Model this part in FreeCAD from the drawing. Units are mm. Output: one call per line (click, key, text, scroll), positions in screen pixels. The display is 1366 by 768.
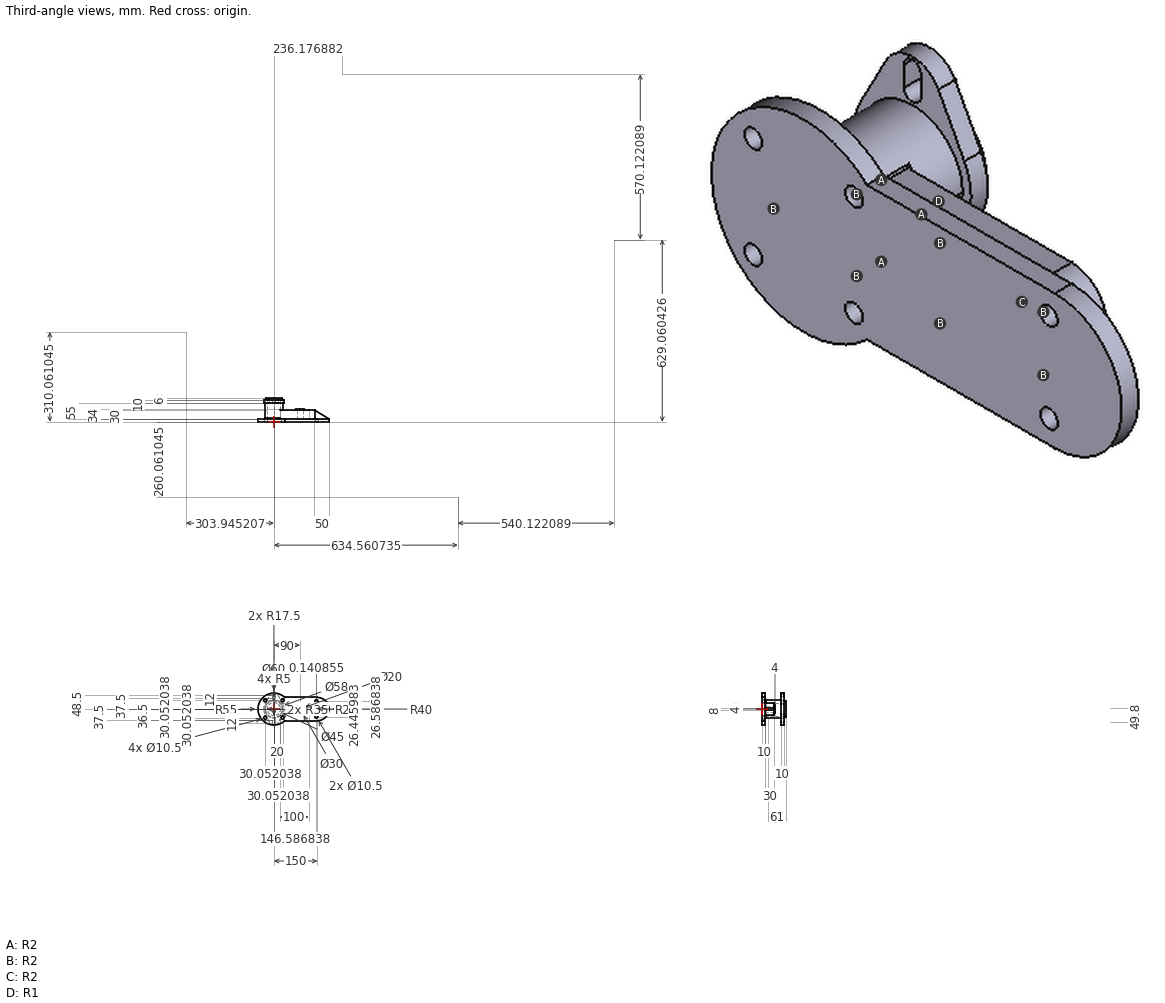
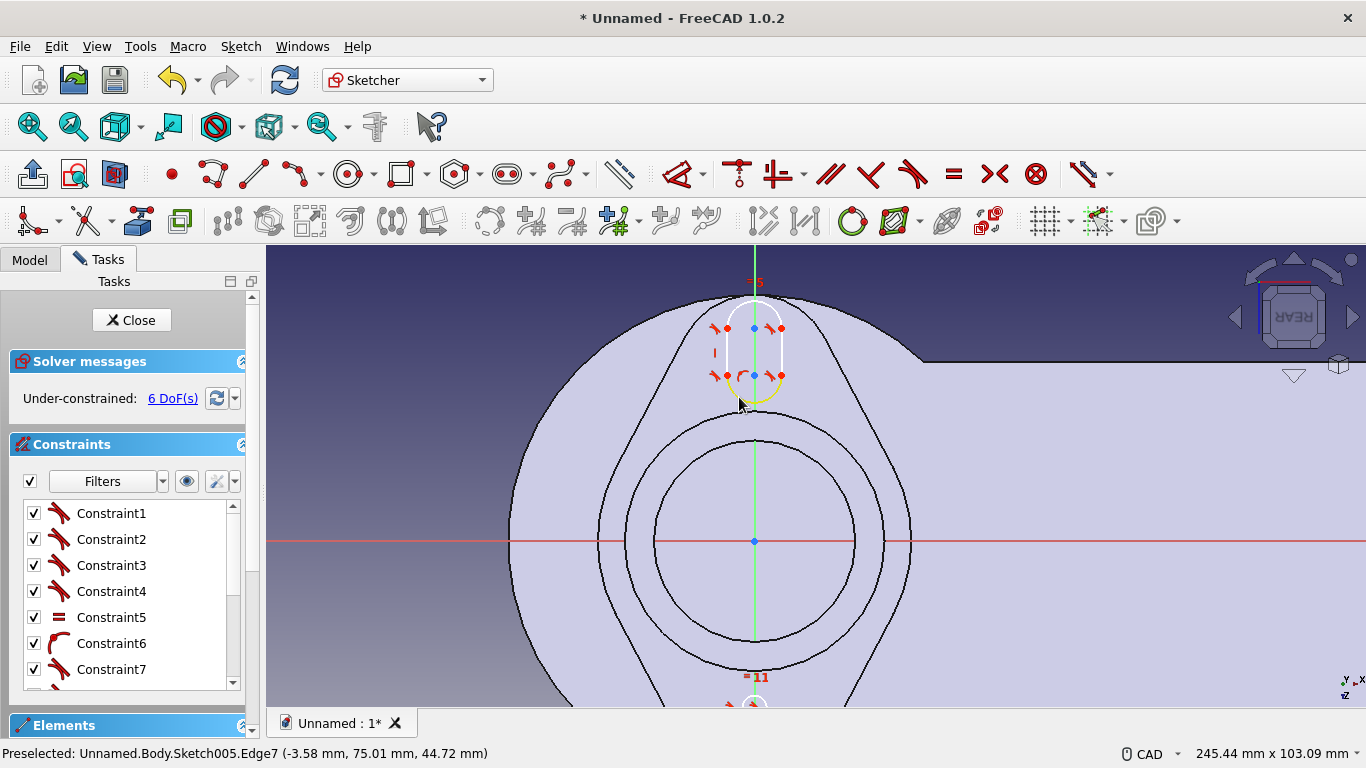
click(739, 398)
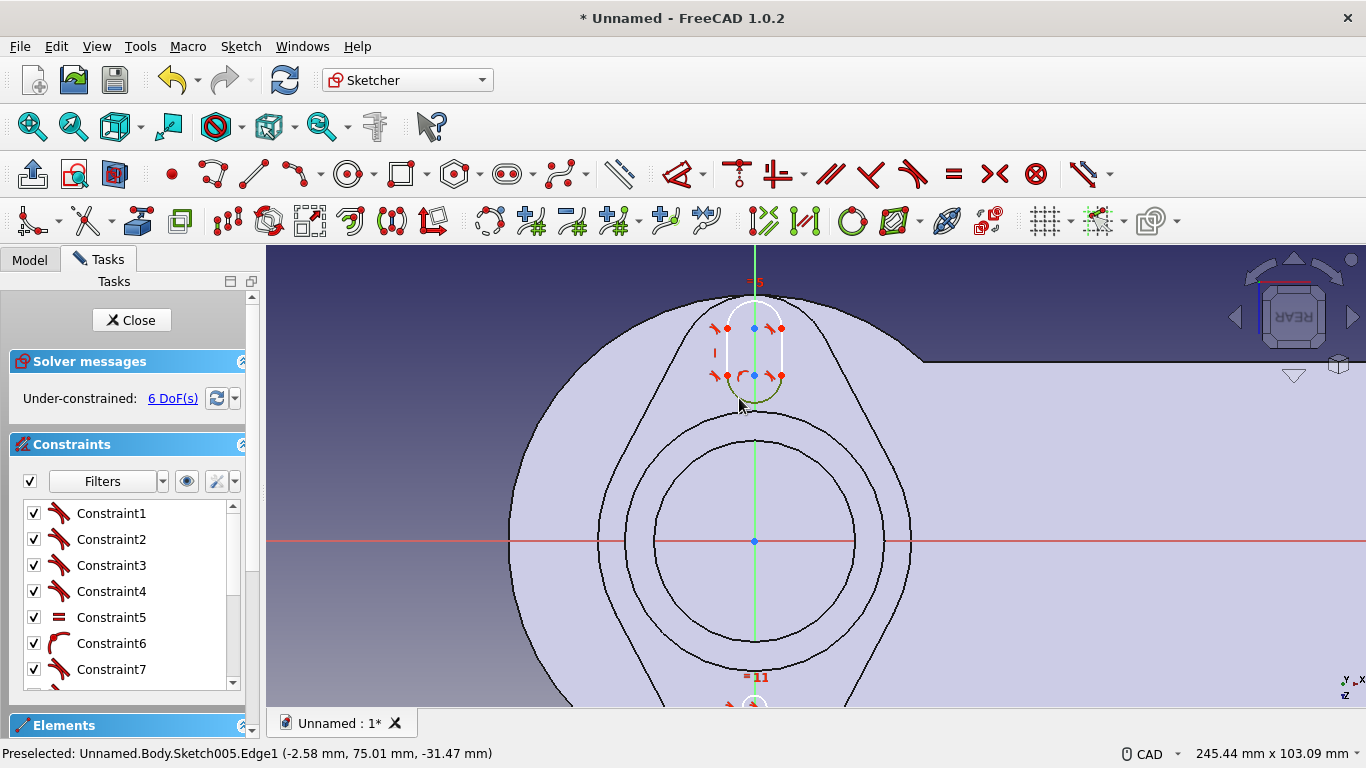
scroll(739, 397, down, 3)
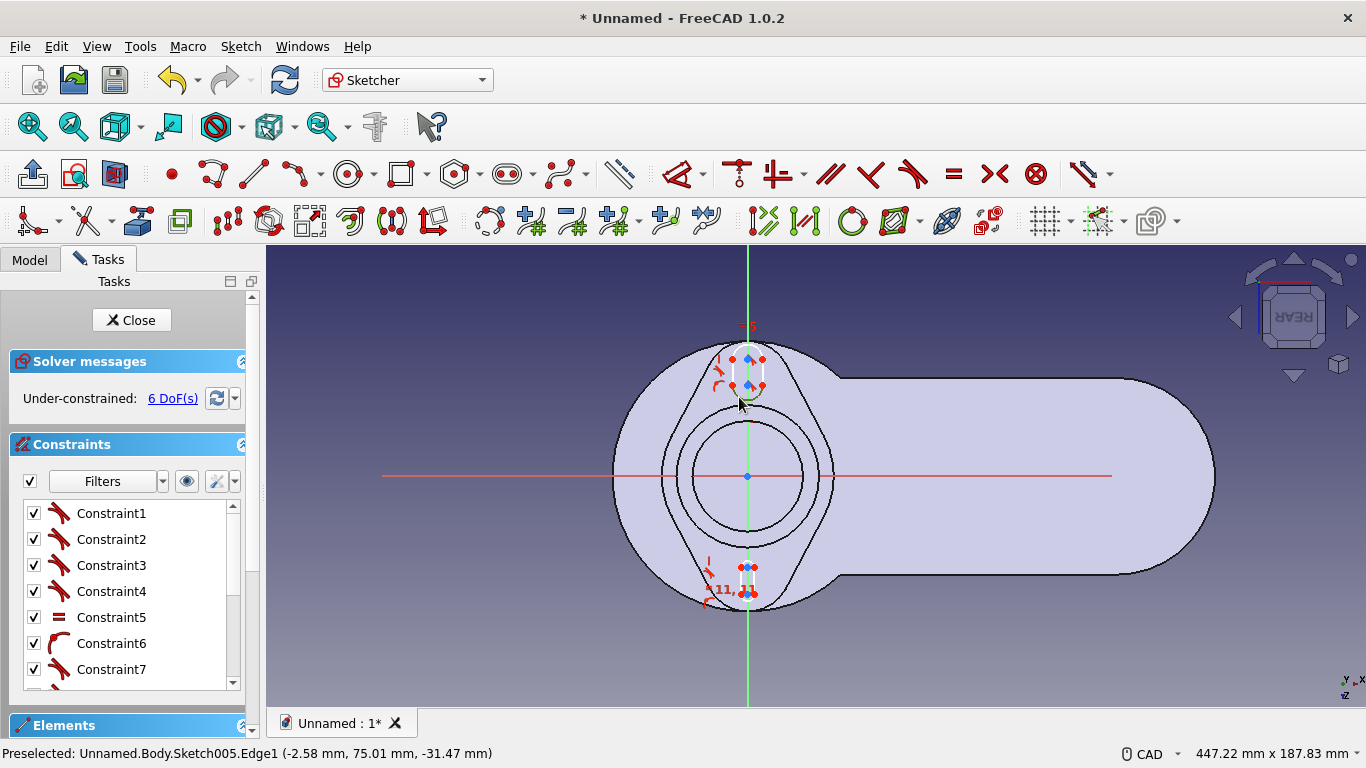
scroll(748, 601, up, 4)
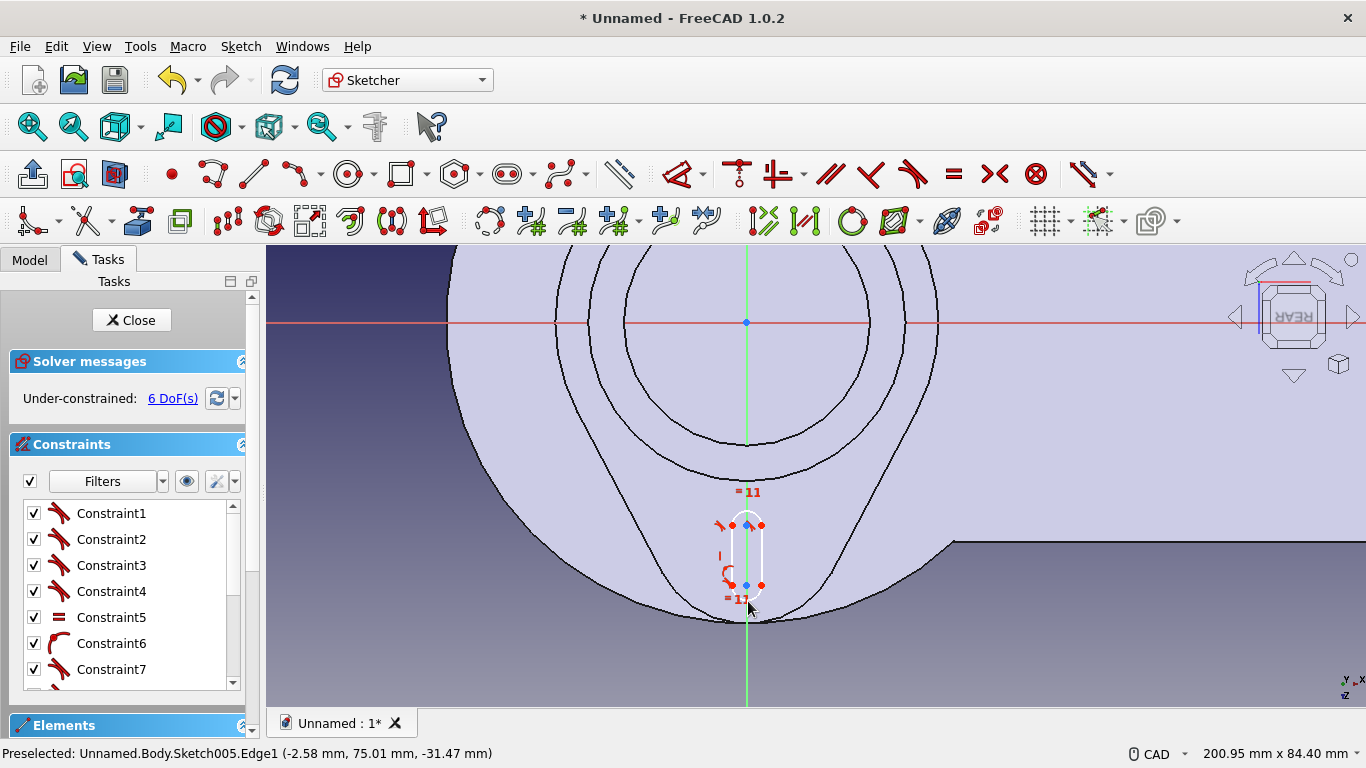
click(759, 594)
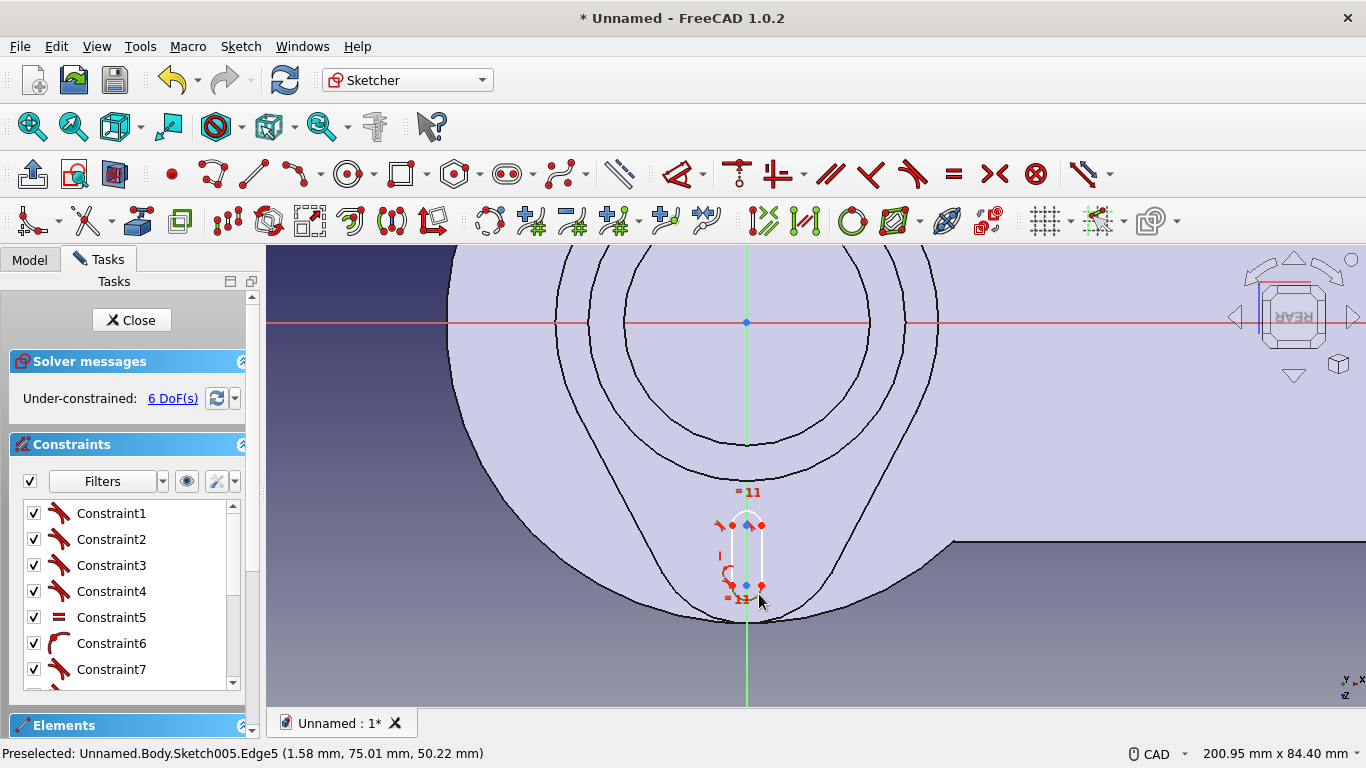
click(954, 174)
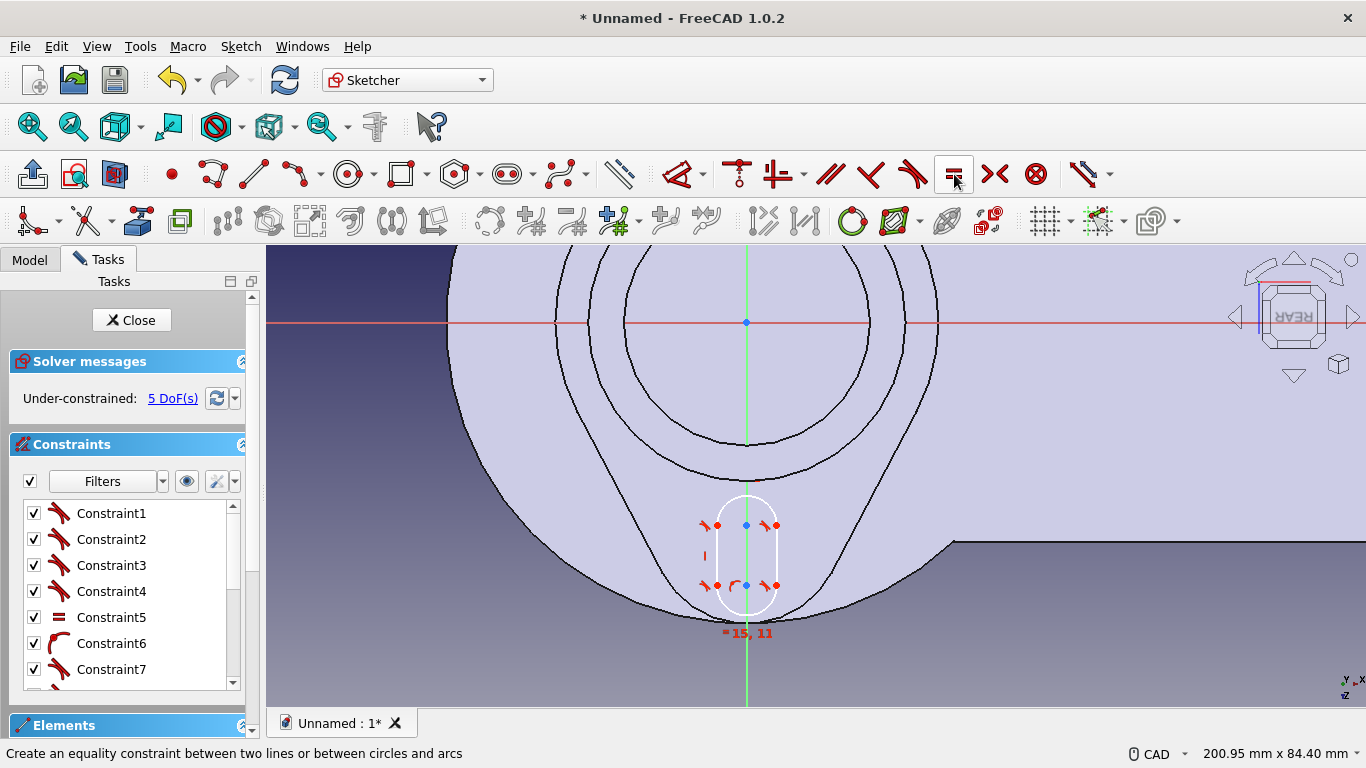
key(d)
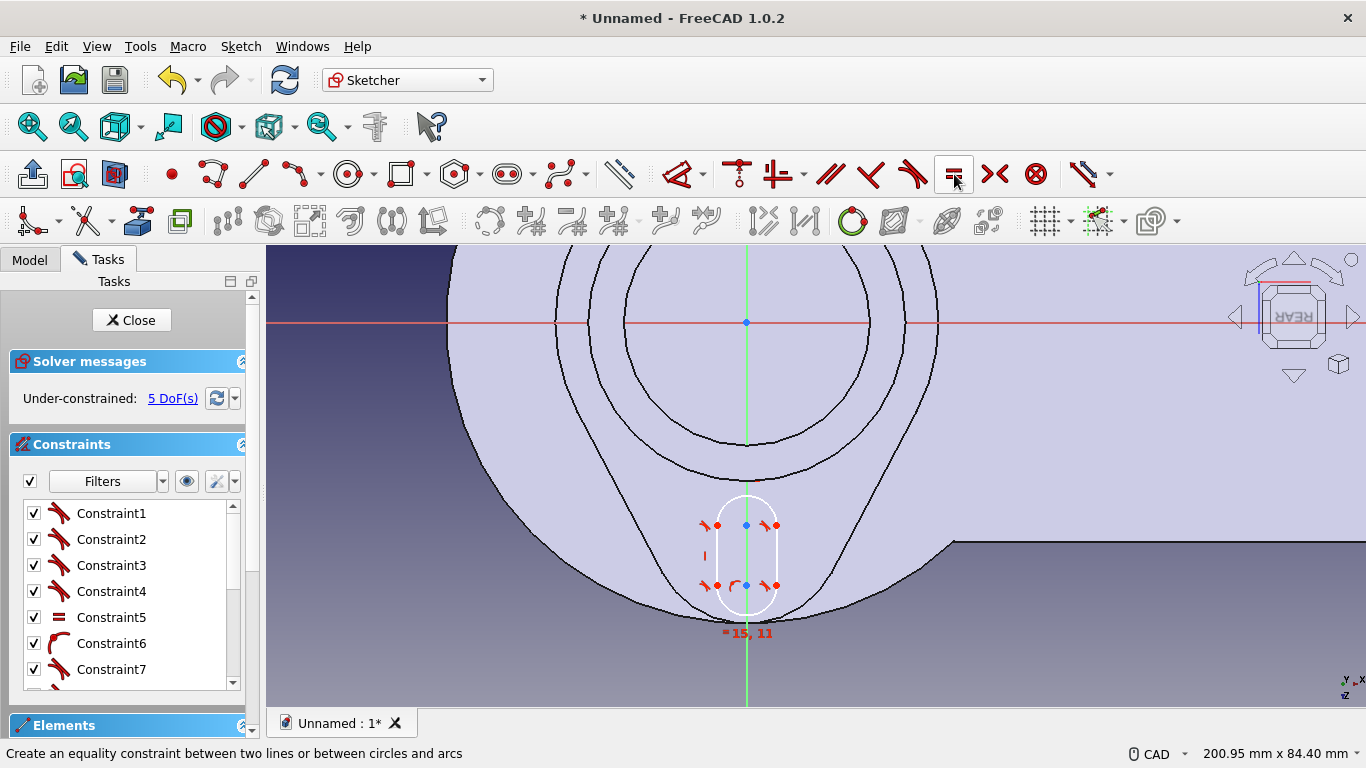
scroll(748, 601, down, 4)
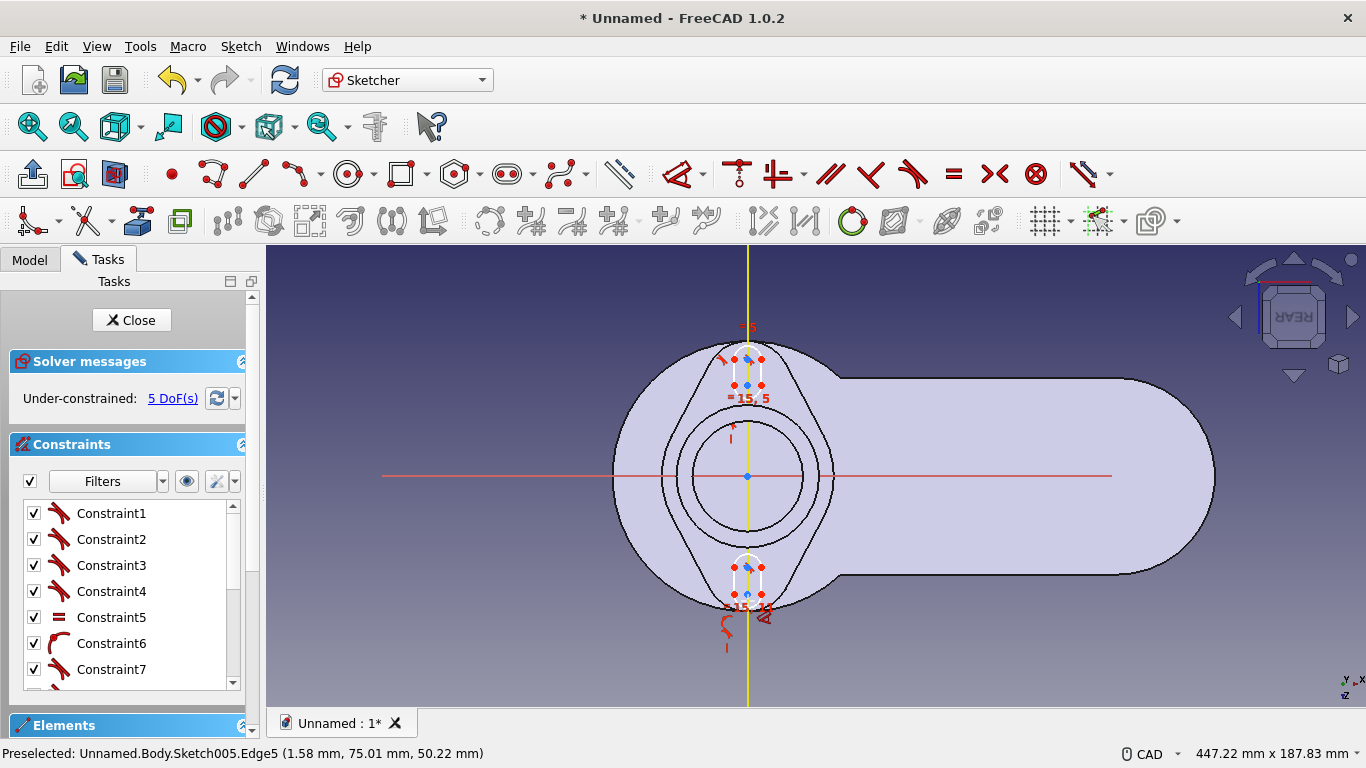
scroll(740, 396, up, 6)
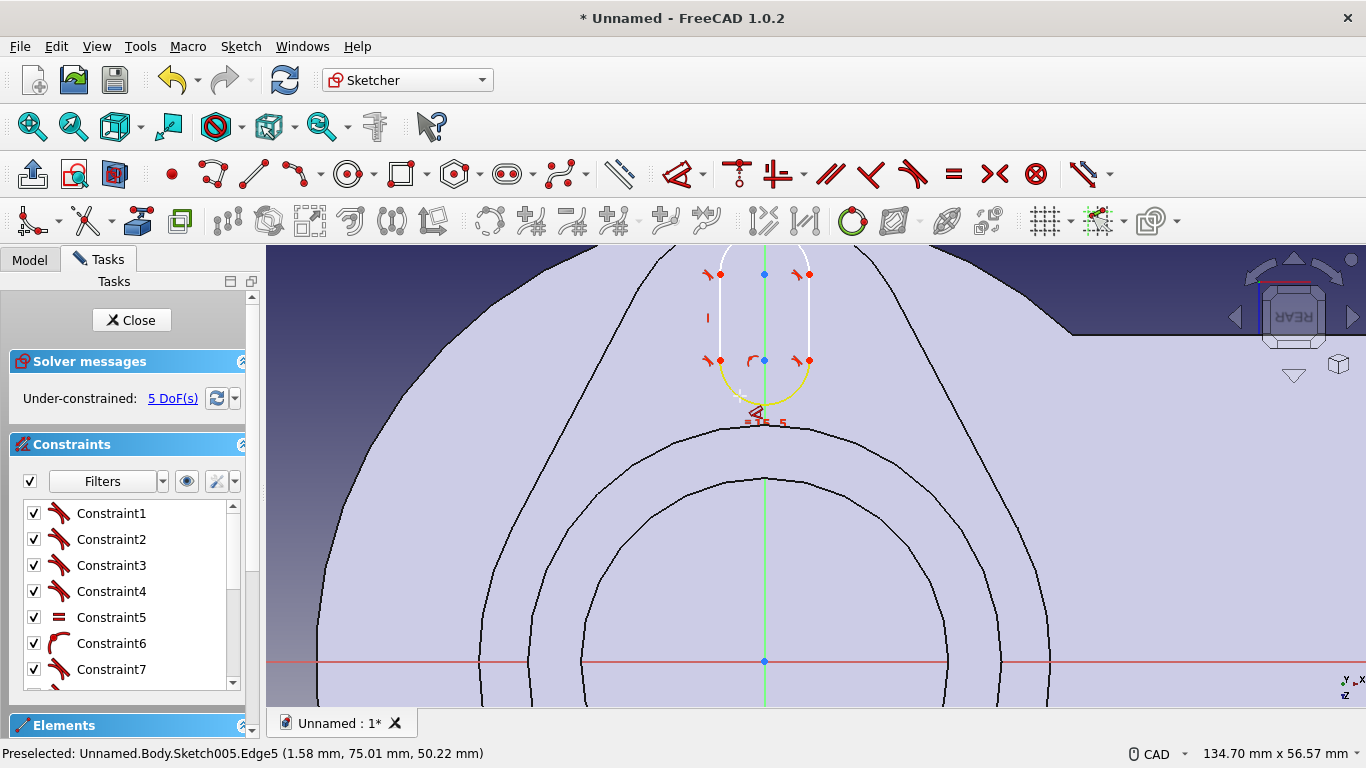
click(739, 396)
click(720, 422)